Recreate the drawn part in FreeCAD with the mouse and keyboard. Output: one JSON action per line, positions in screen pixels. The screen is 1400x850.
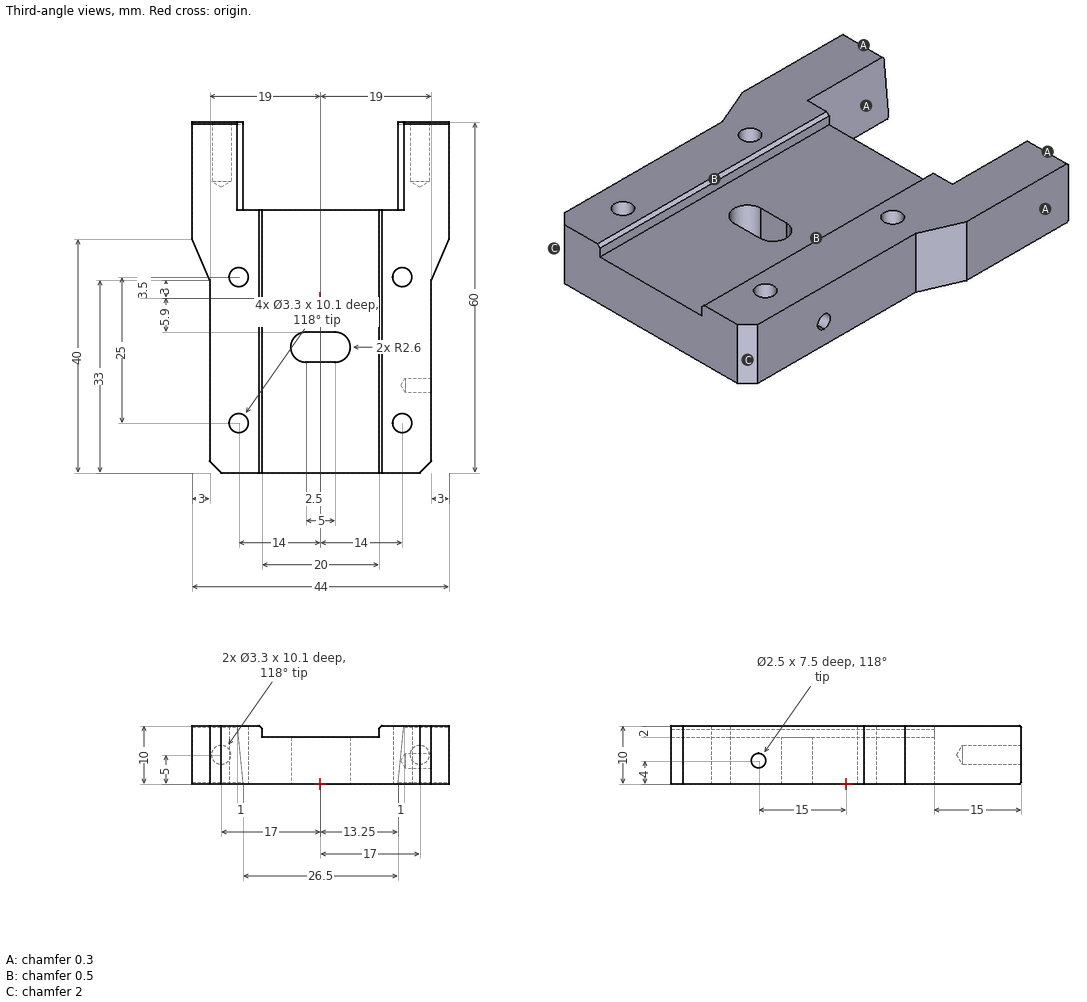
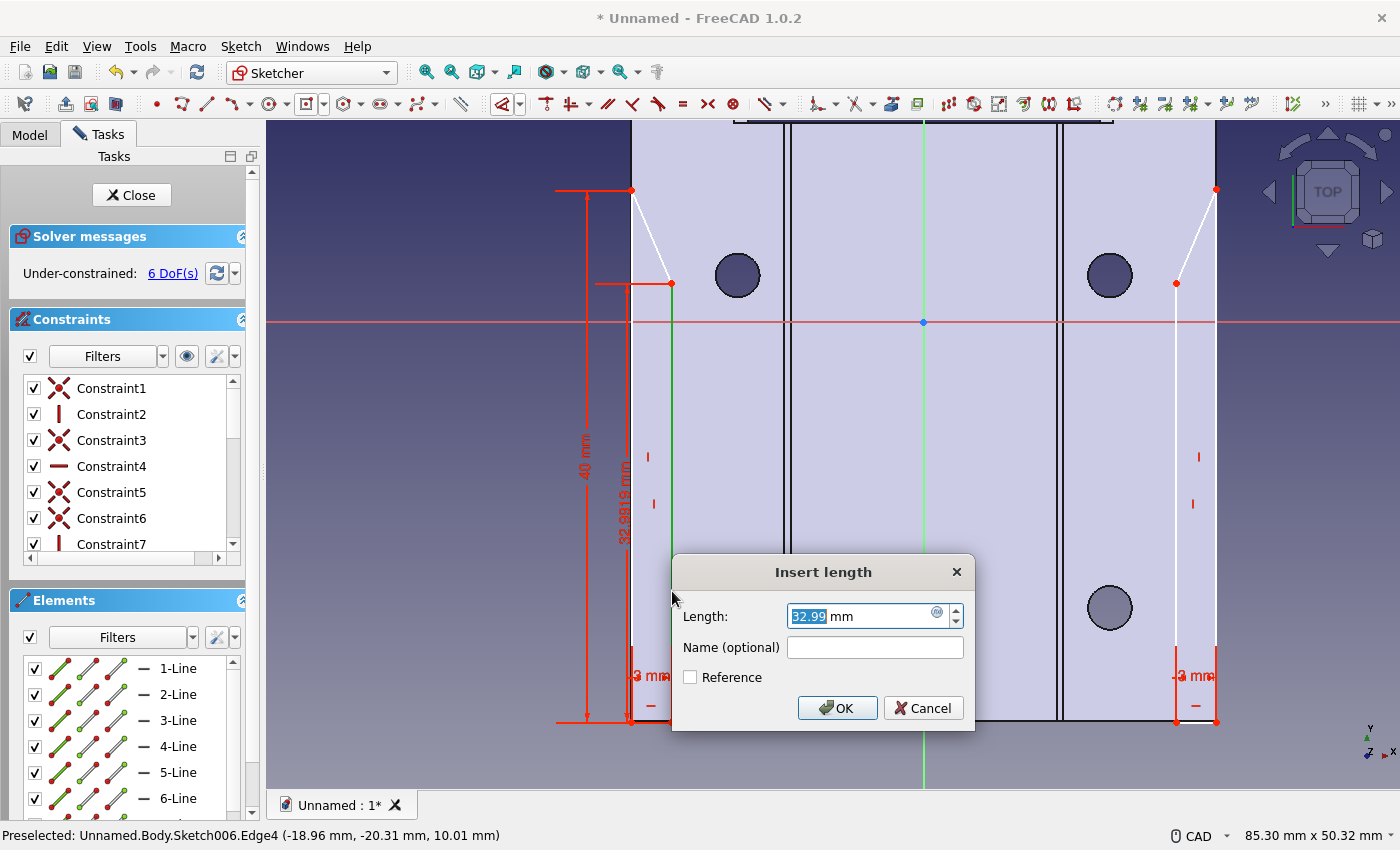
{"action": "type", "text": "33"}
{"action": "key", "text": "Return"}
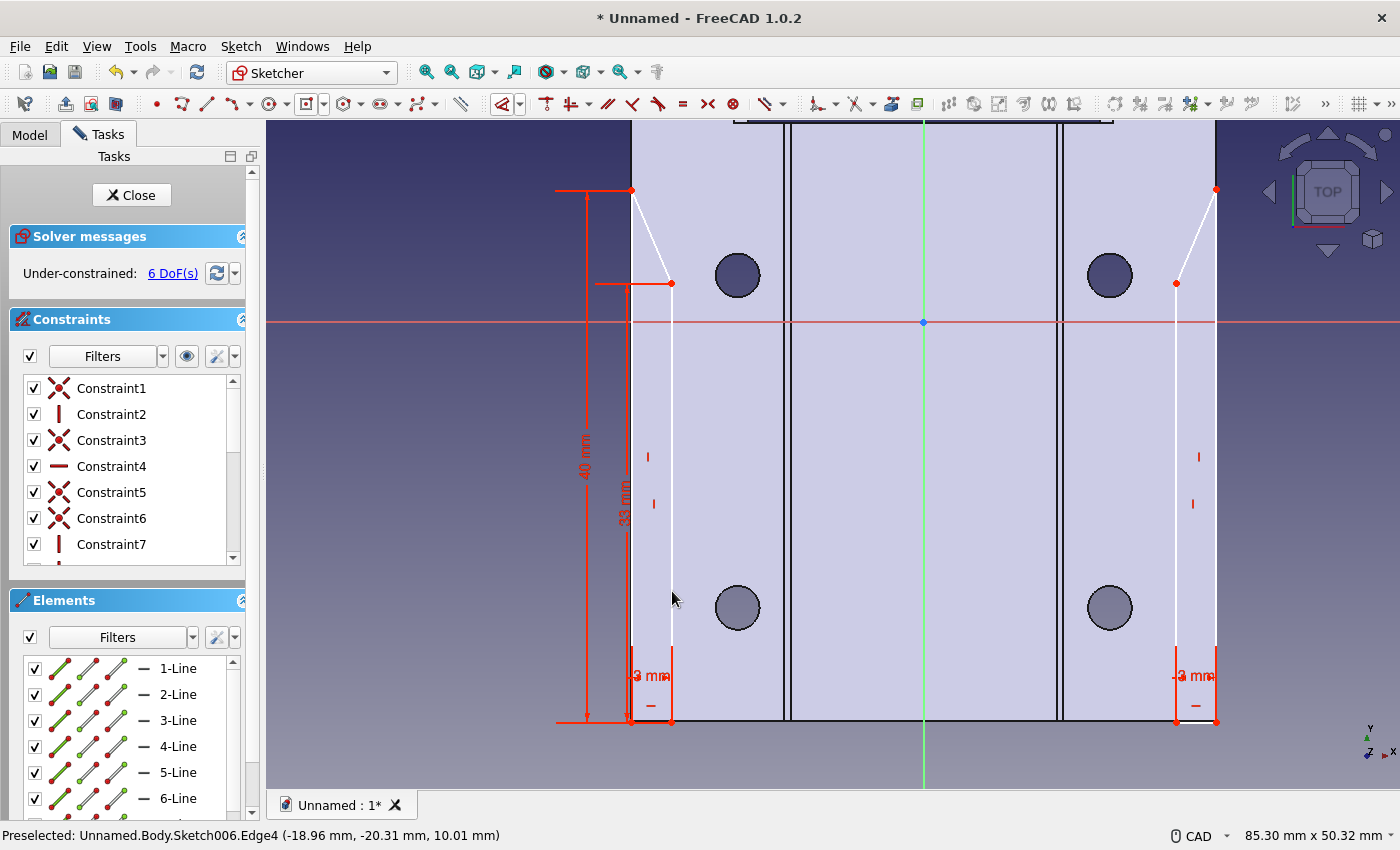
{"action": "left_click", "coordinate": [1176, 416]}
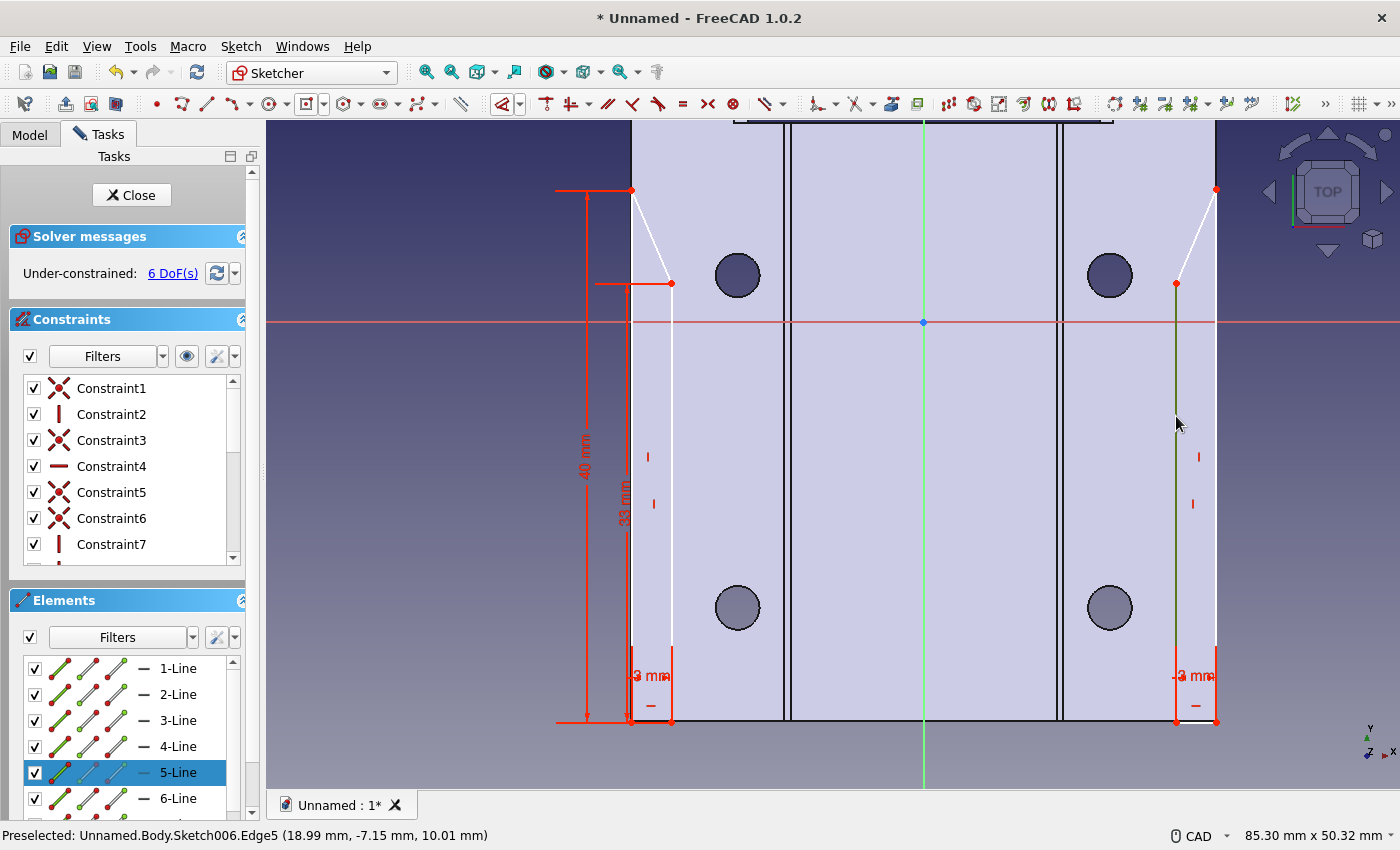
{"action": "left_click", "coordinate": [520, 104]}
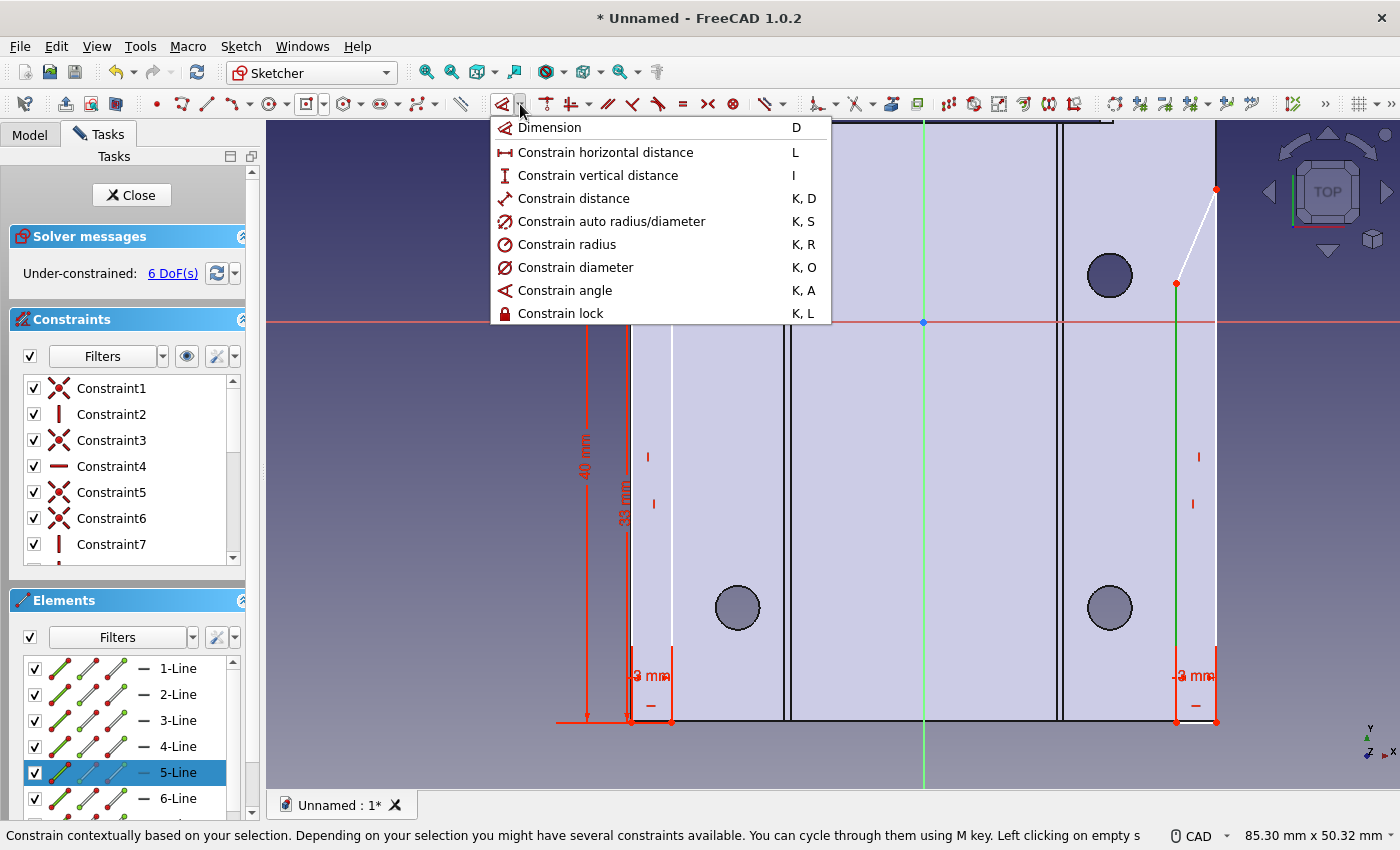
{"action": "left_click", "coordinate": [661, 176]}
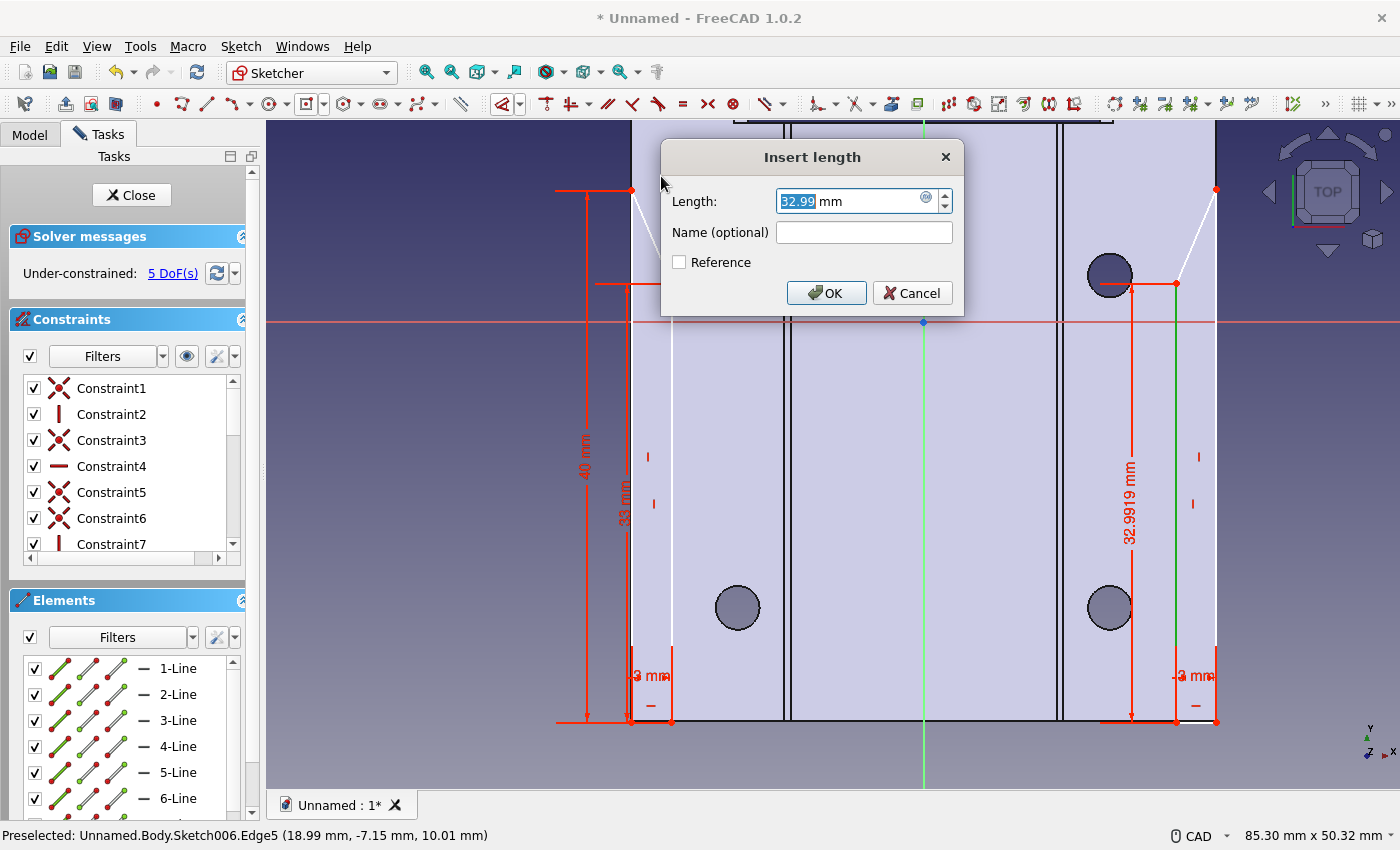
{"action": "type", "text": "33"}
{"action": "key", "text": "Return"}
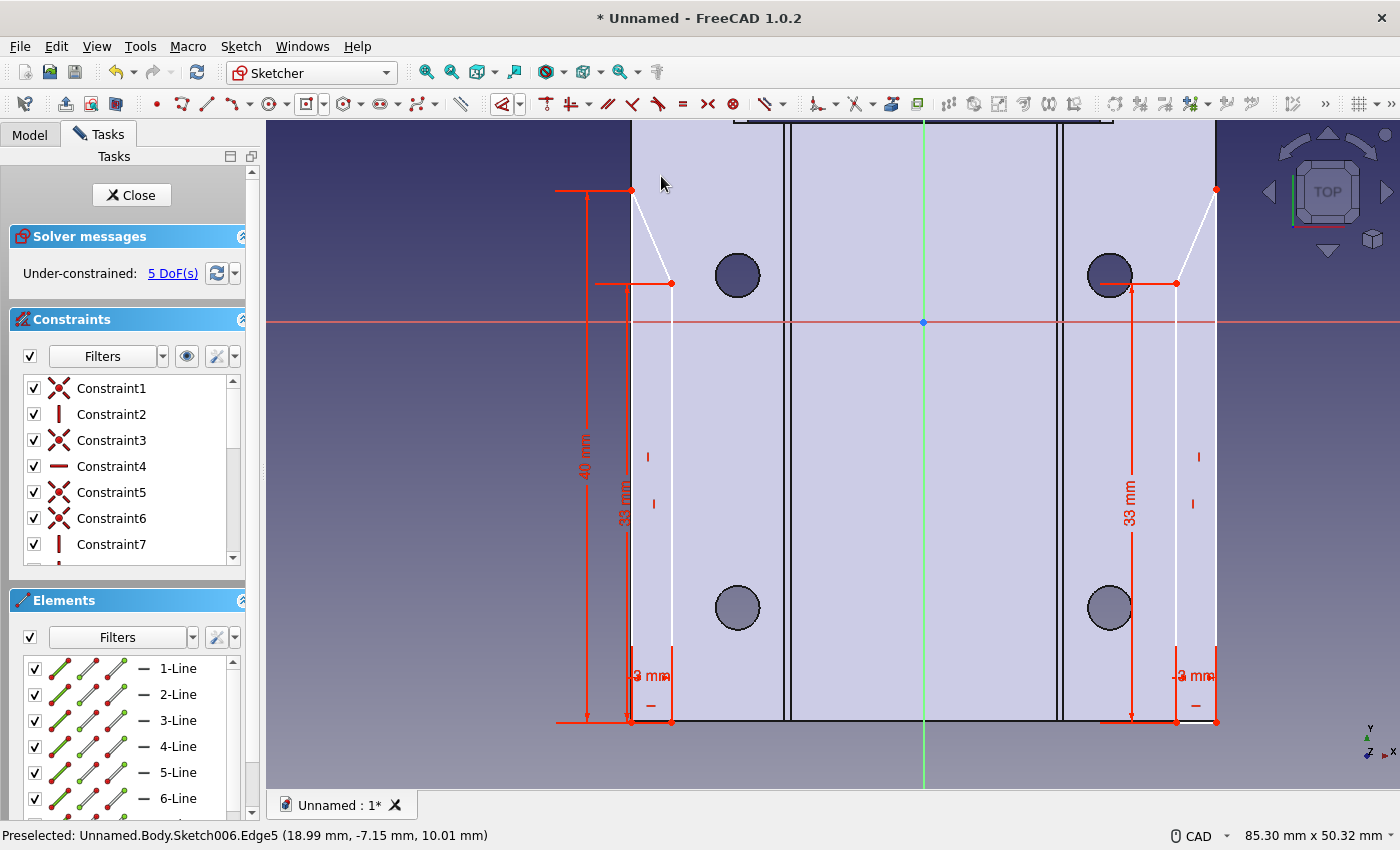
{"action": "left_click", "coordinate": [1216, 563]}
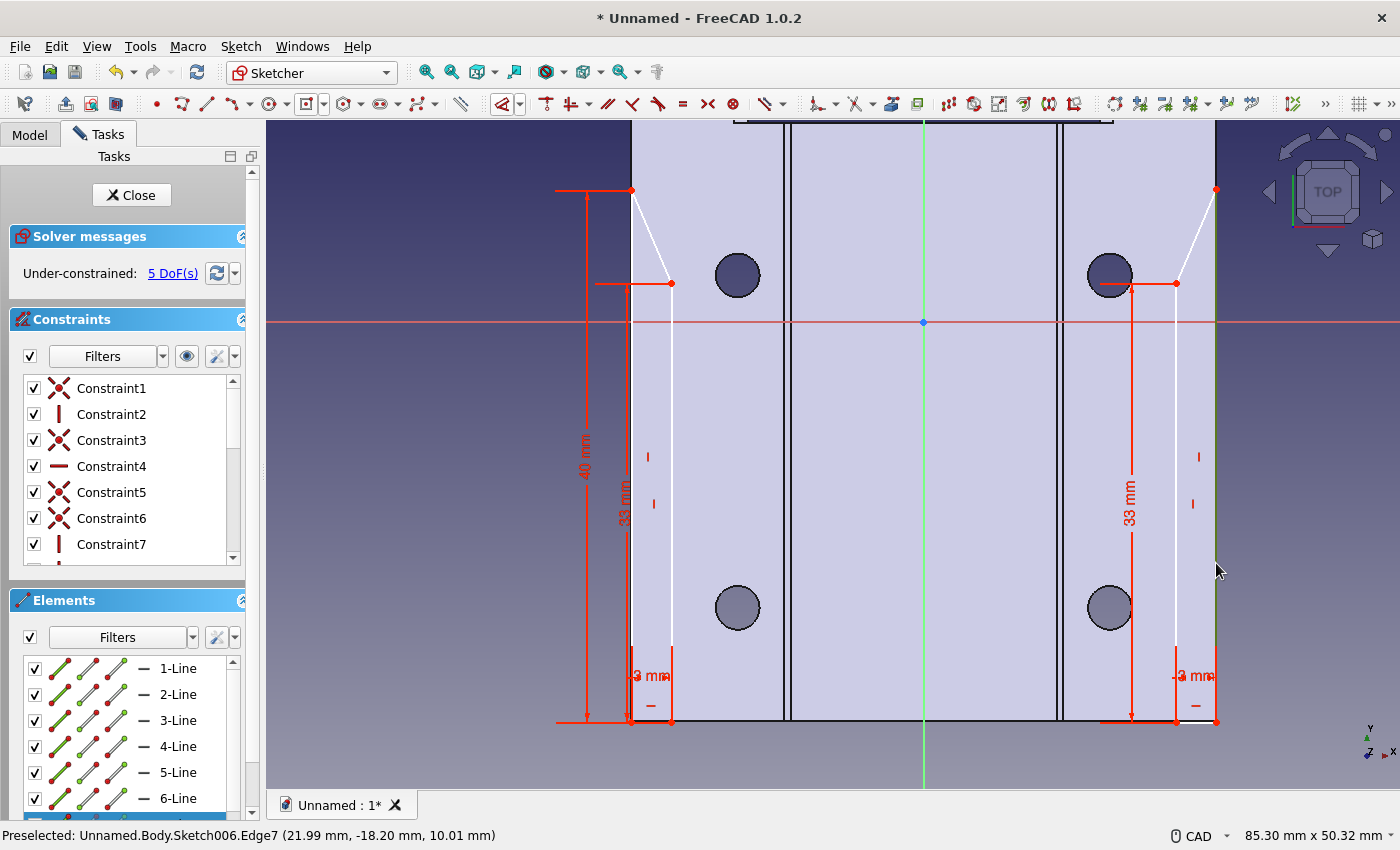
{"action": "key", "text": "i"}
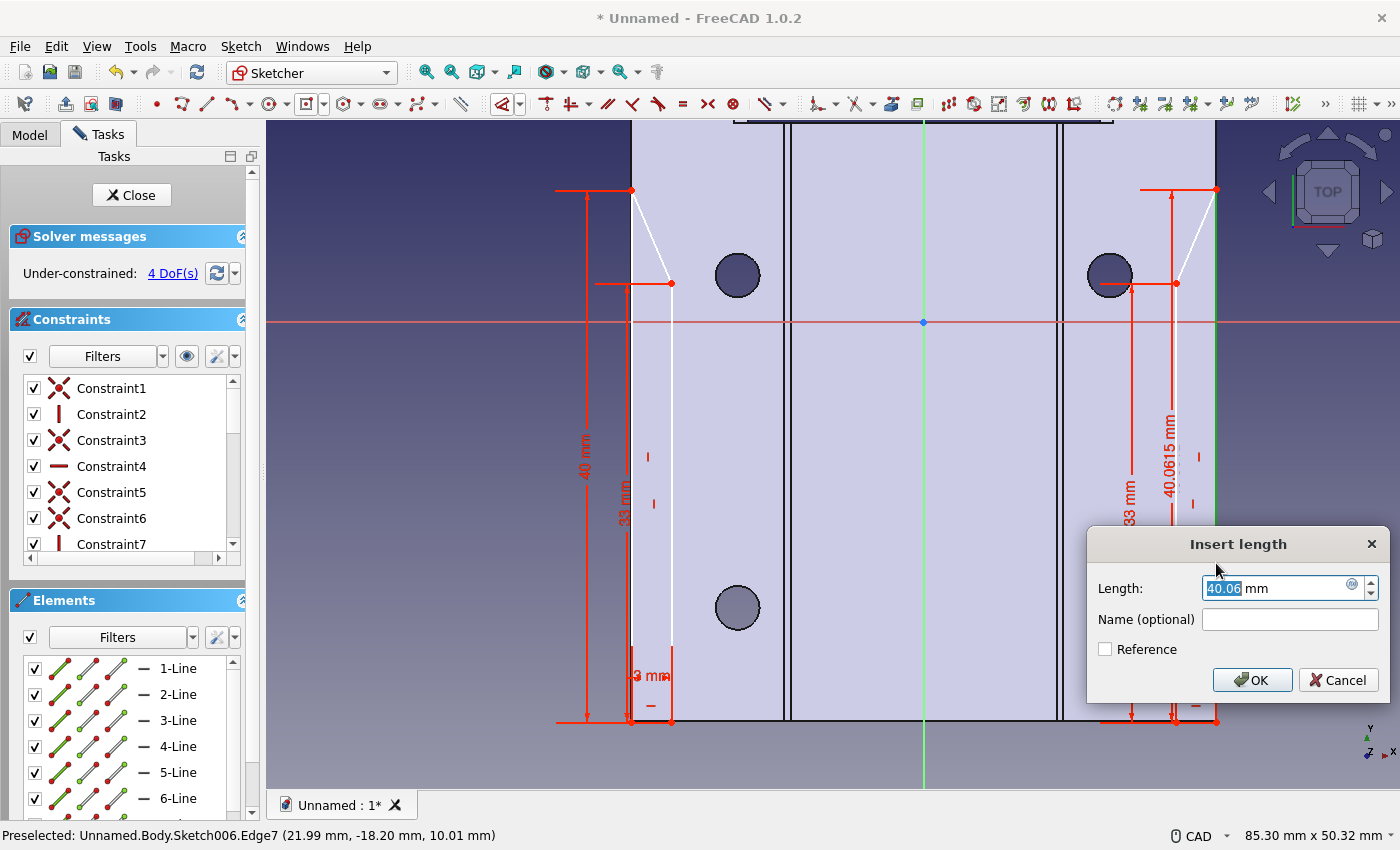
{"action": "type", "text": "40"}
{"action": "key", "text": "Return"}